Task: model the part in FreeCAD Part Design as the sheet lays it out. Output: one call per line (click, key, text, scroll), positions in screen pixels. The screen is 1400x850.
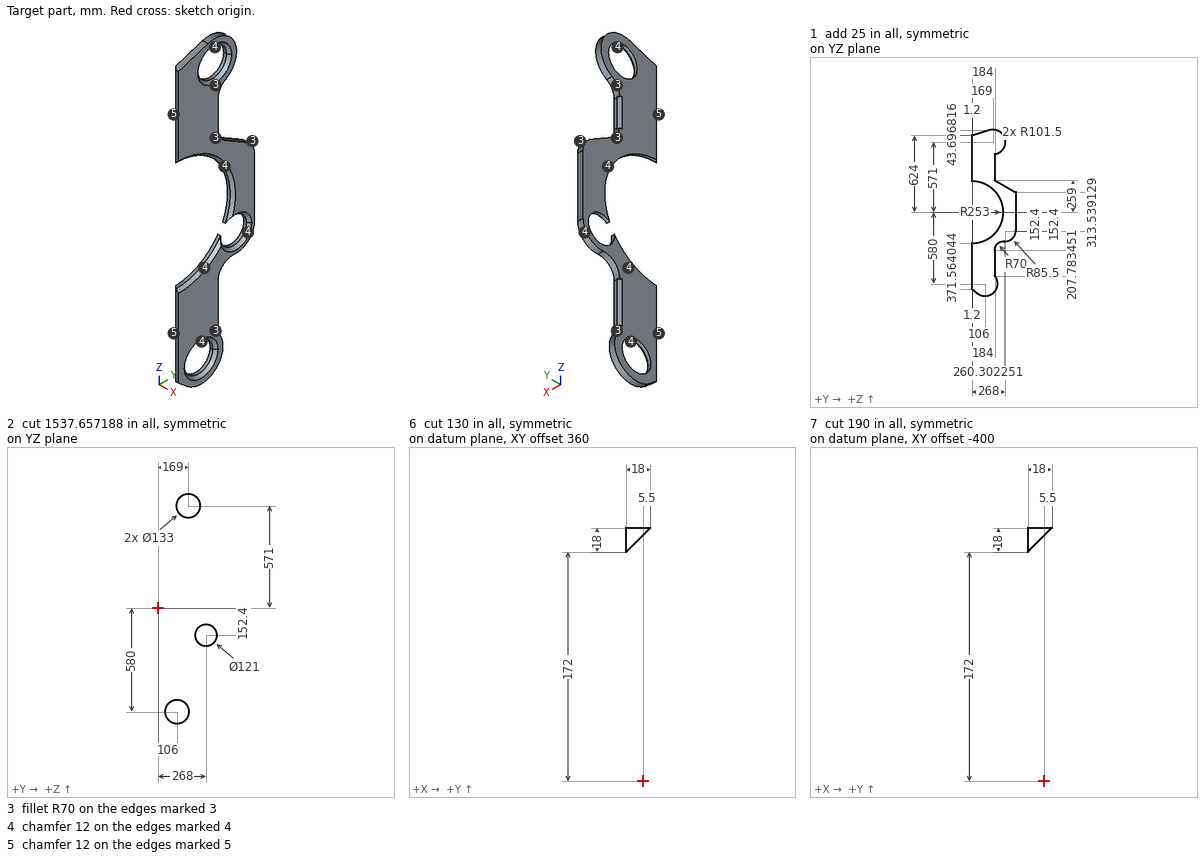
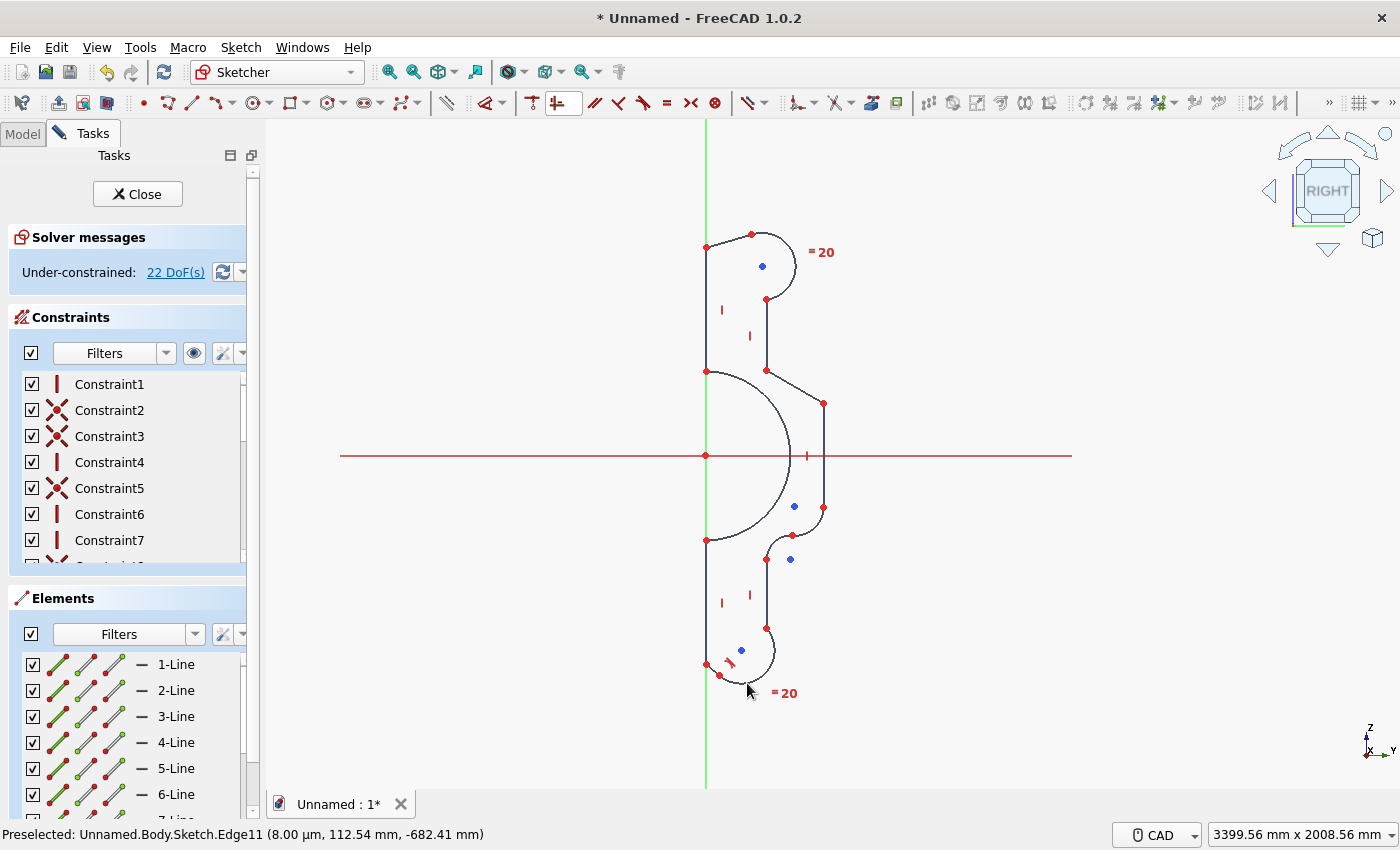
key(d)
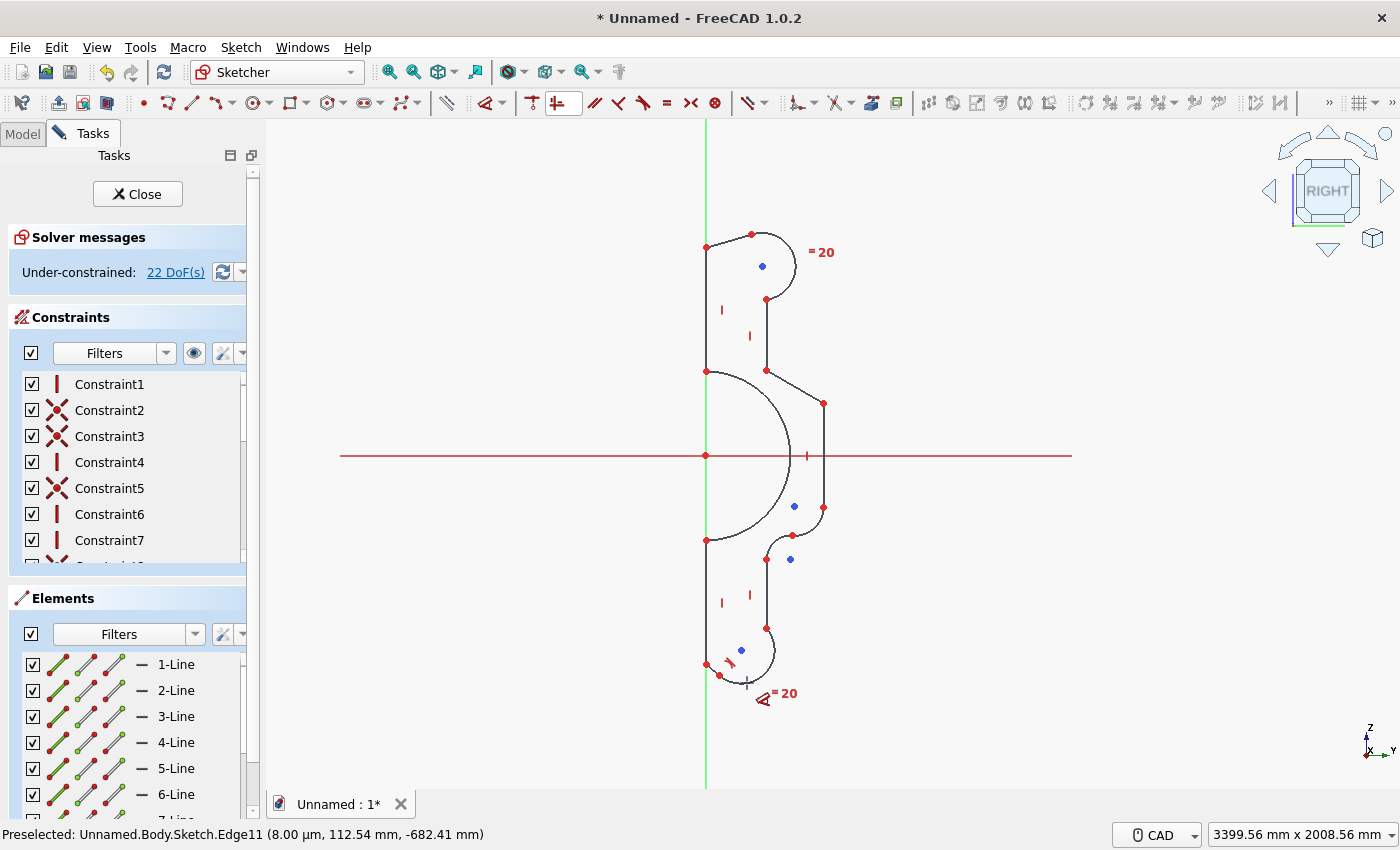
click(792, 281)
click(821, 295)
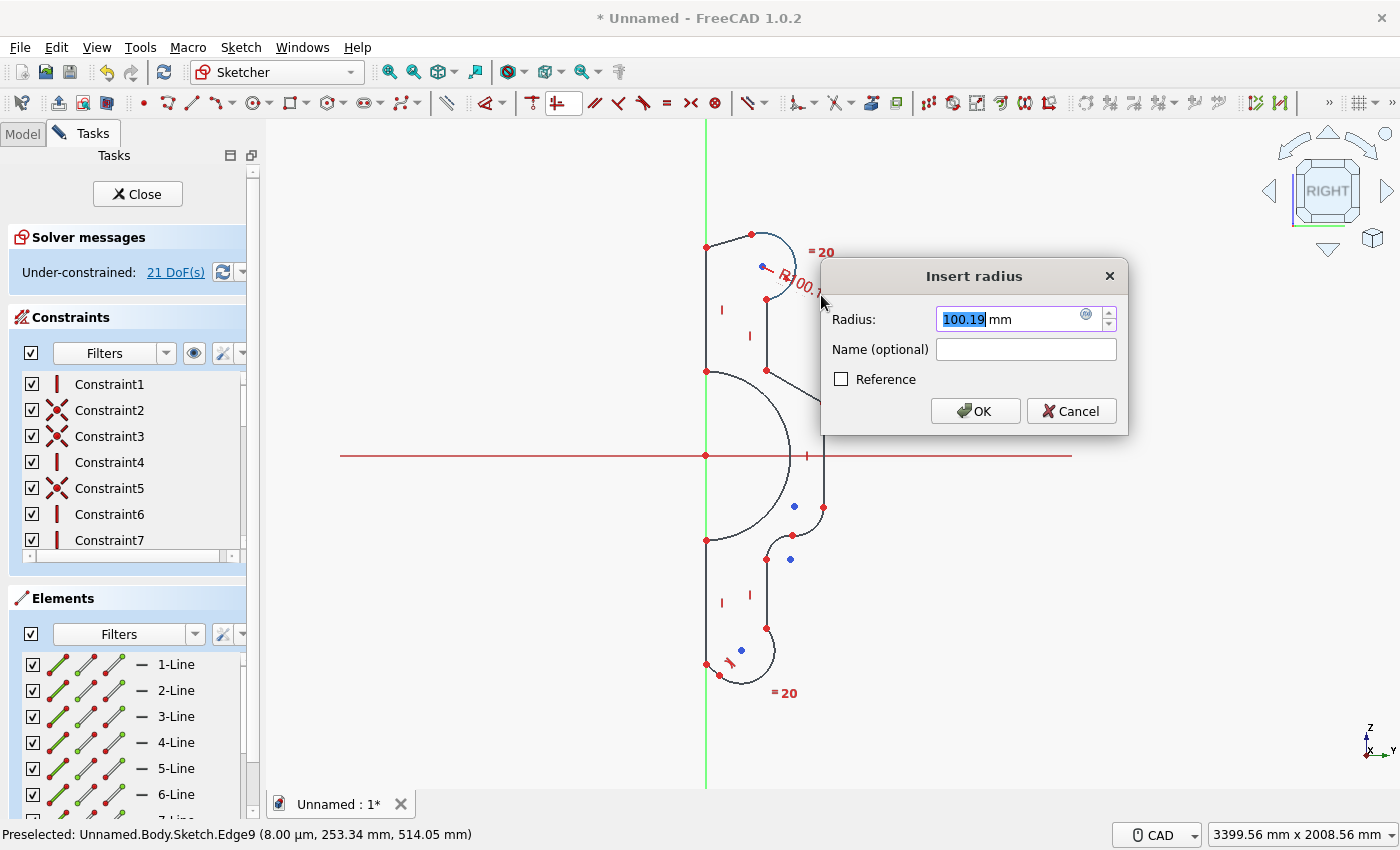
text(101.5)
key(Return)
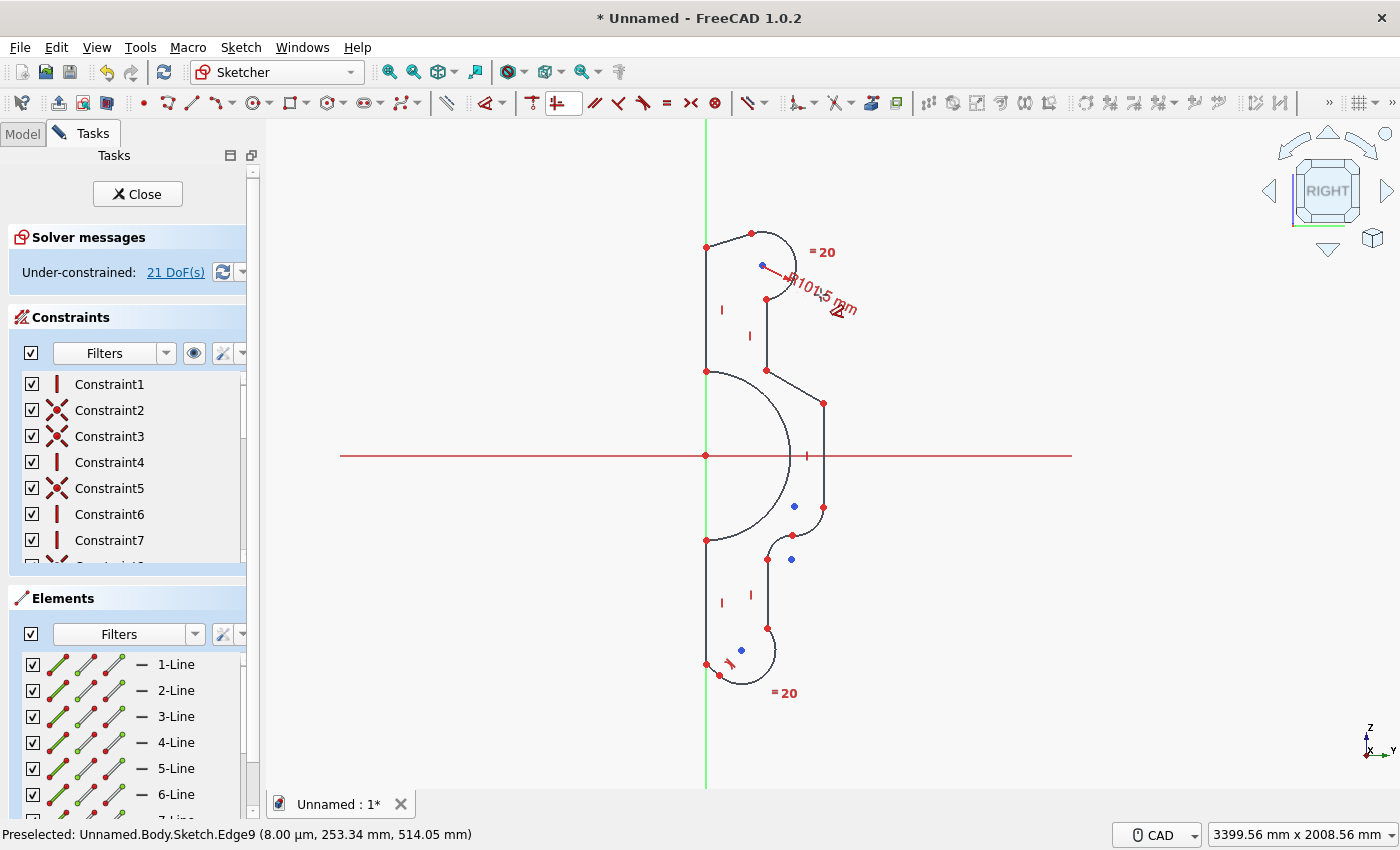
click(774, 505)
click(638, 550)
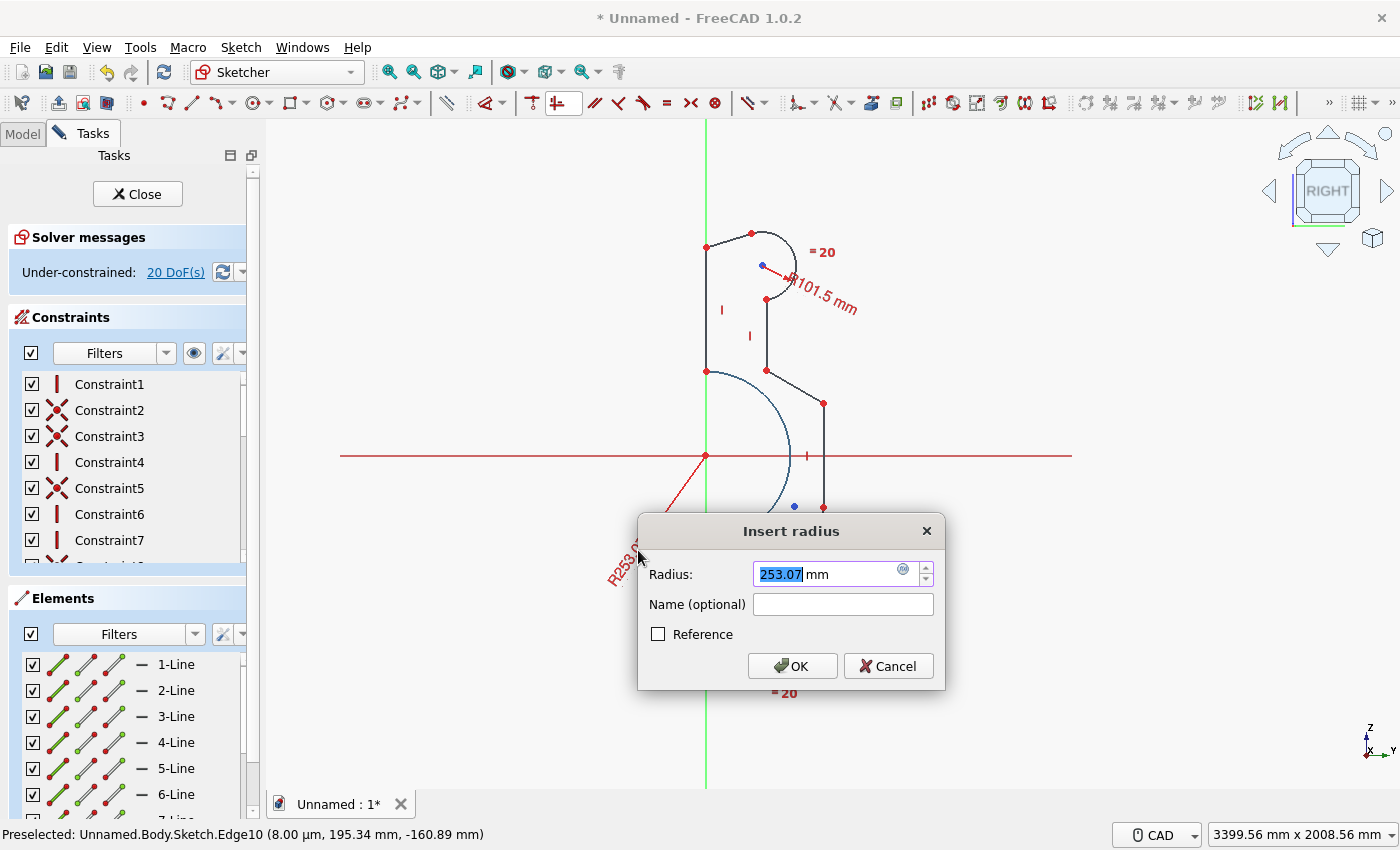
text(253)
key(Return)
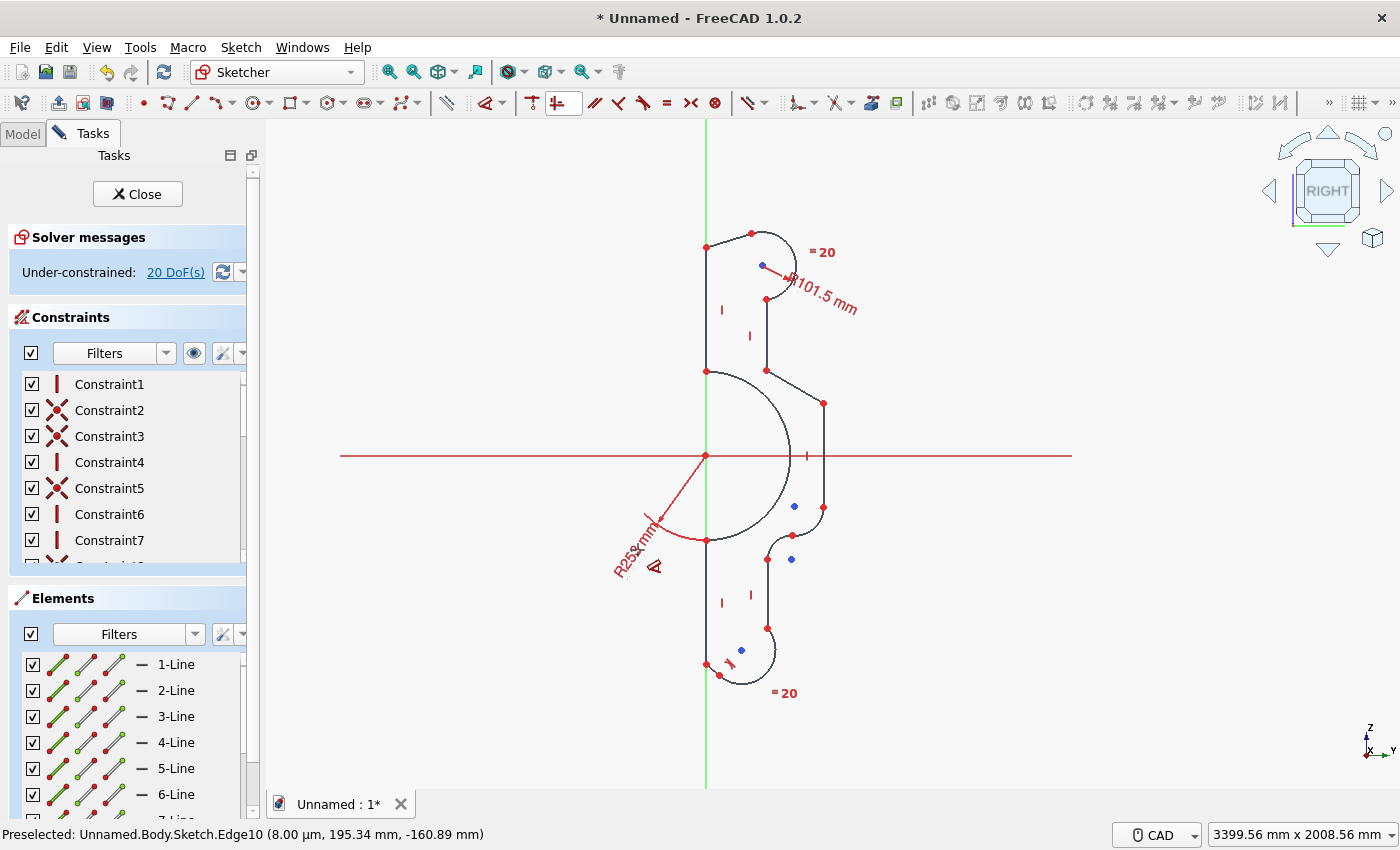
scroll(781, 538, up, 3)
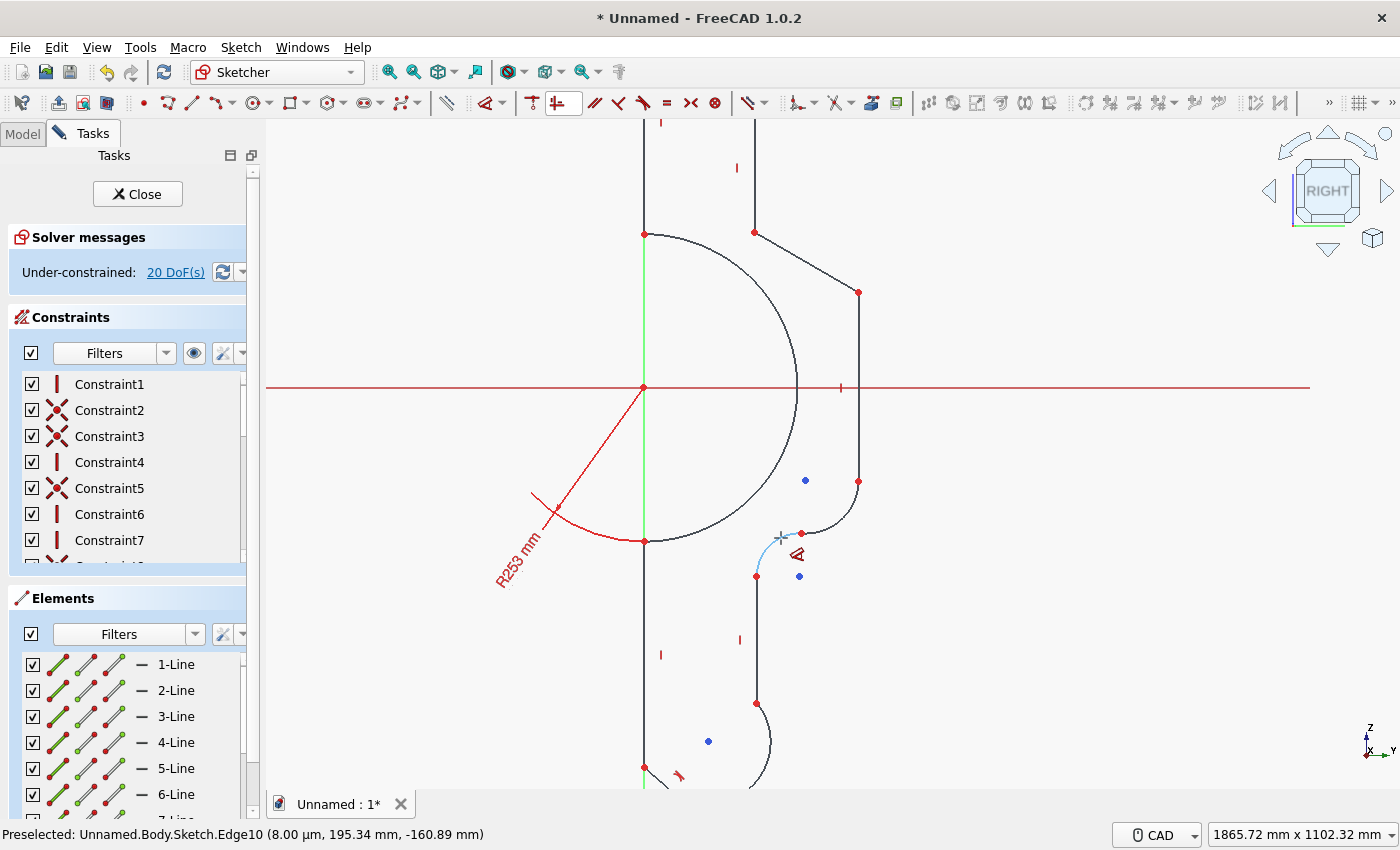
click(781, 537)
click(767, 508)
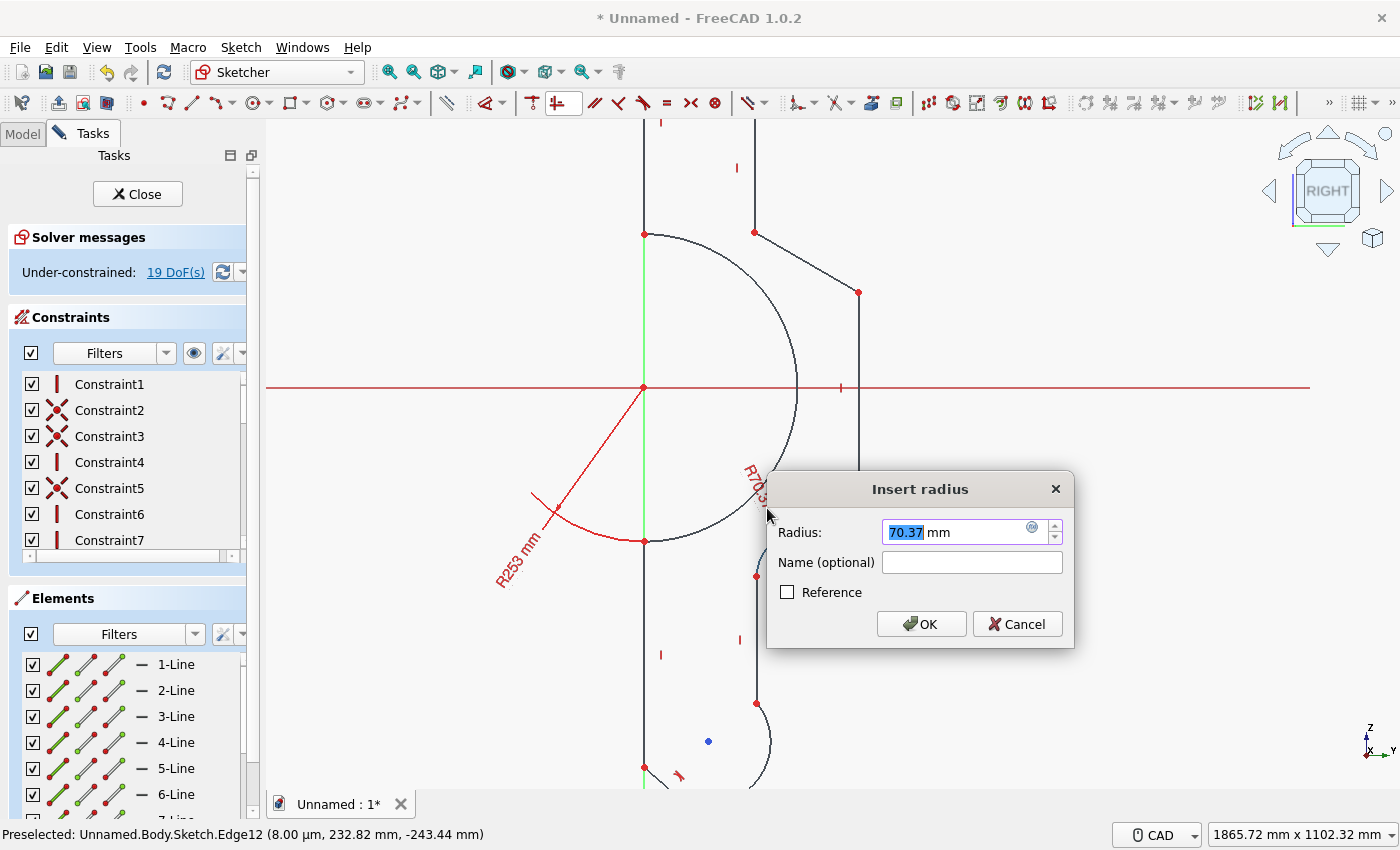
text(70)
key(Return)